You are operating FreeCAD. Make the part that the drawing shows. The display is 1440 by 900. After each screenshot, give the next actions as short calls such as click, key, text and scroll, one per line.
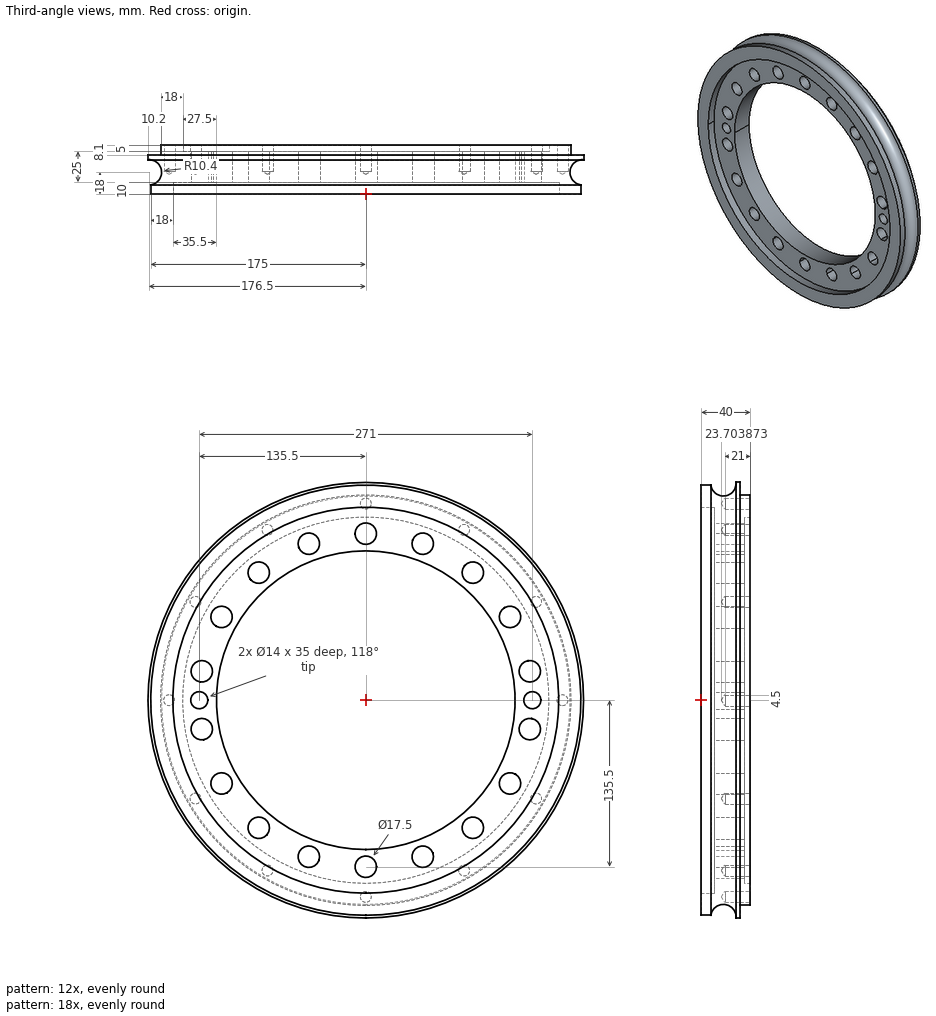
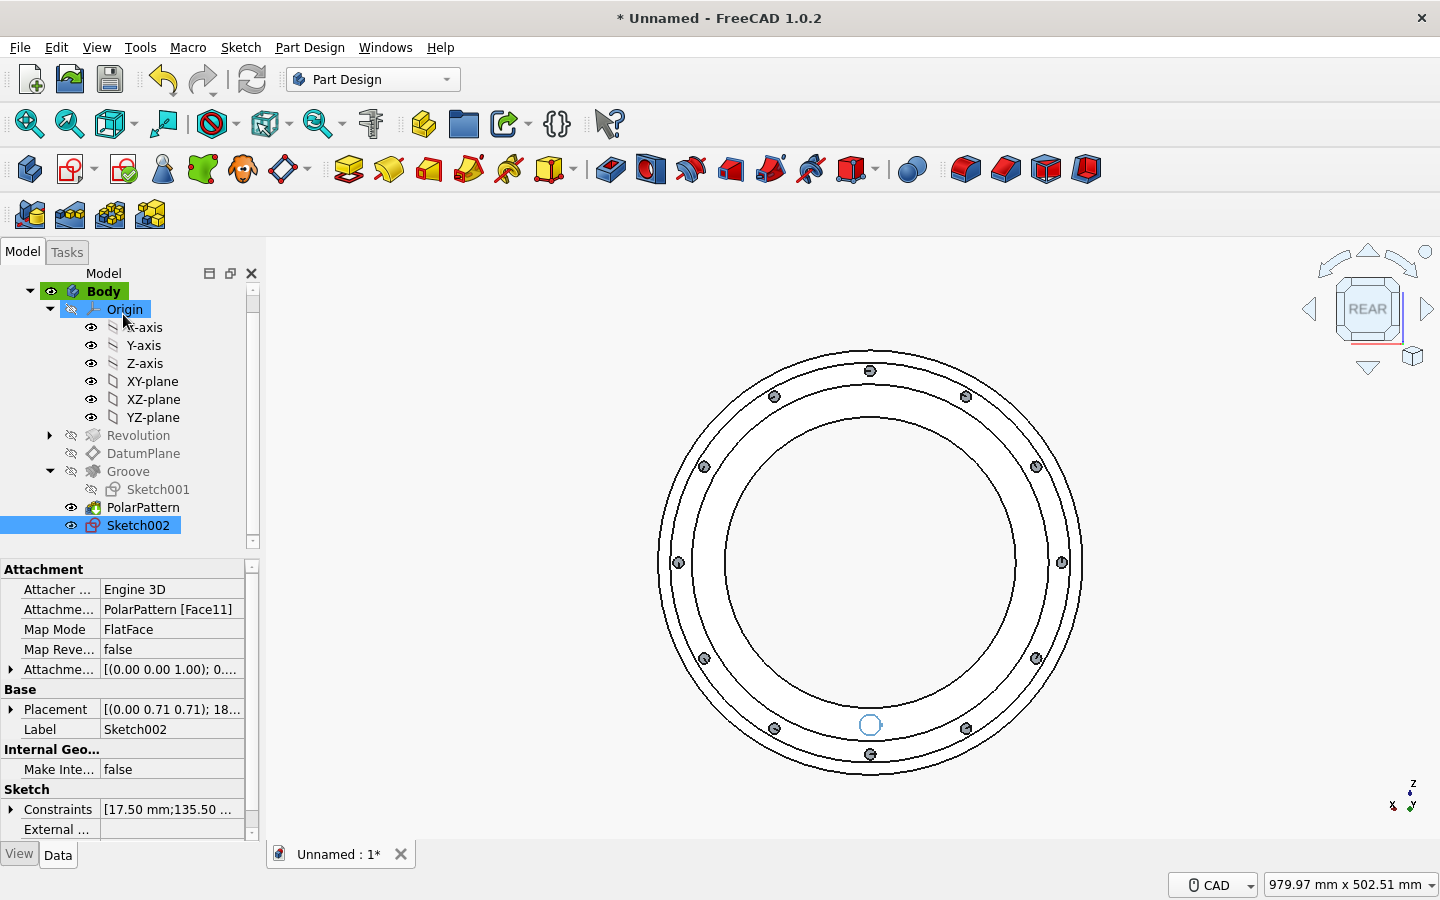
click(612, 170)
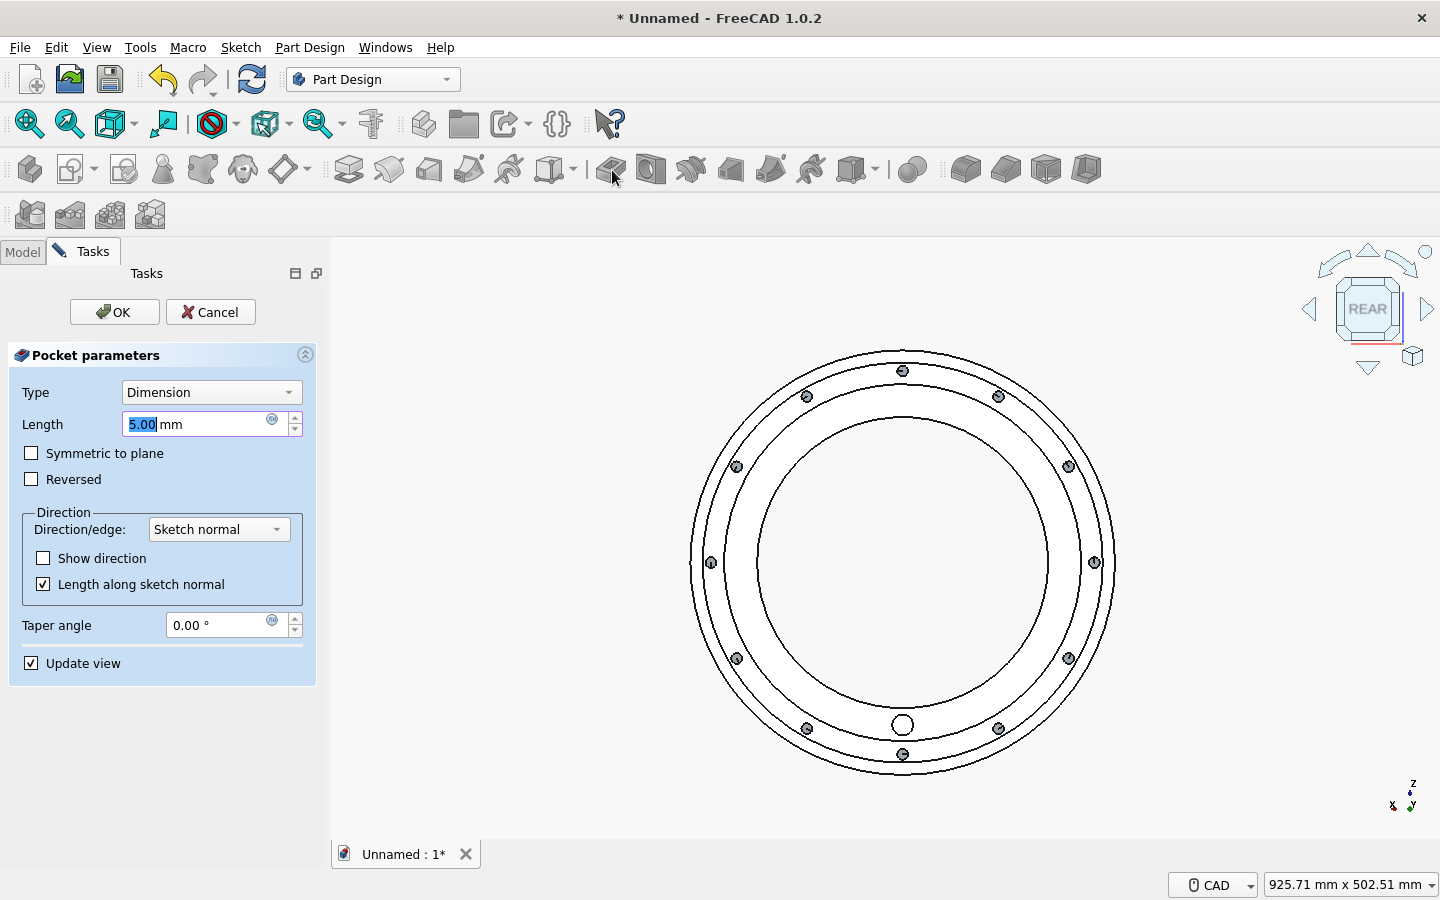
click(212, 392)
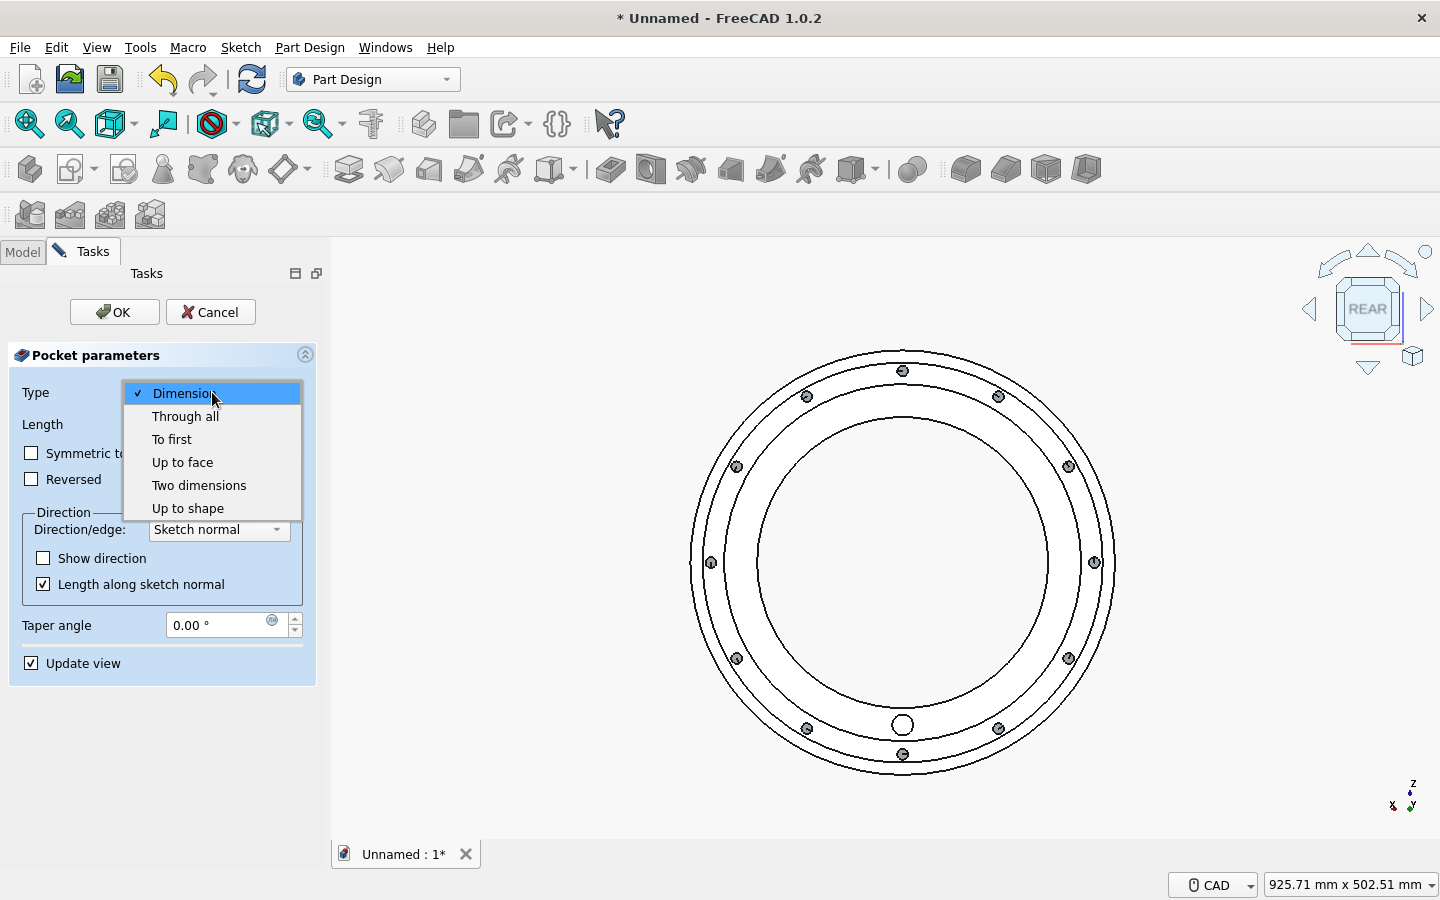
click(212, 416)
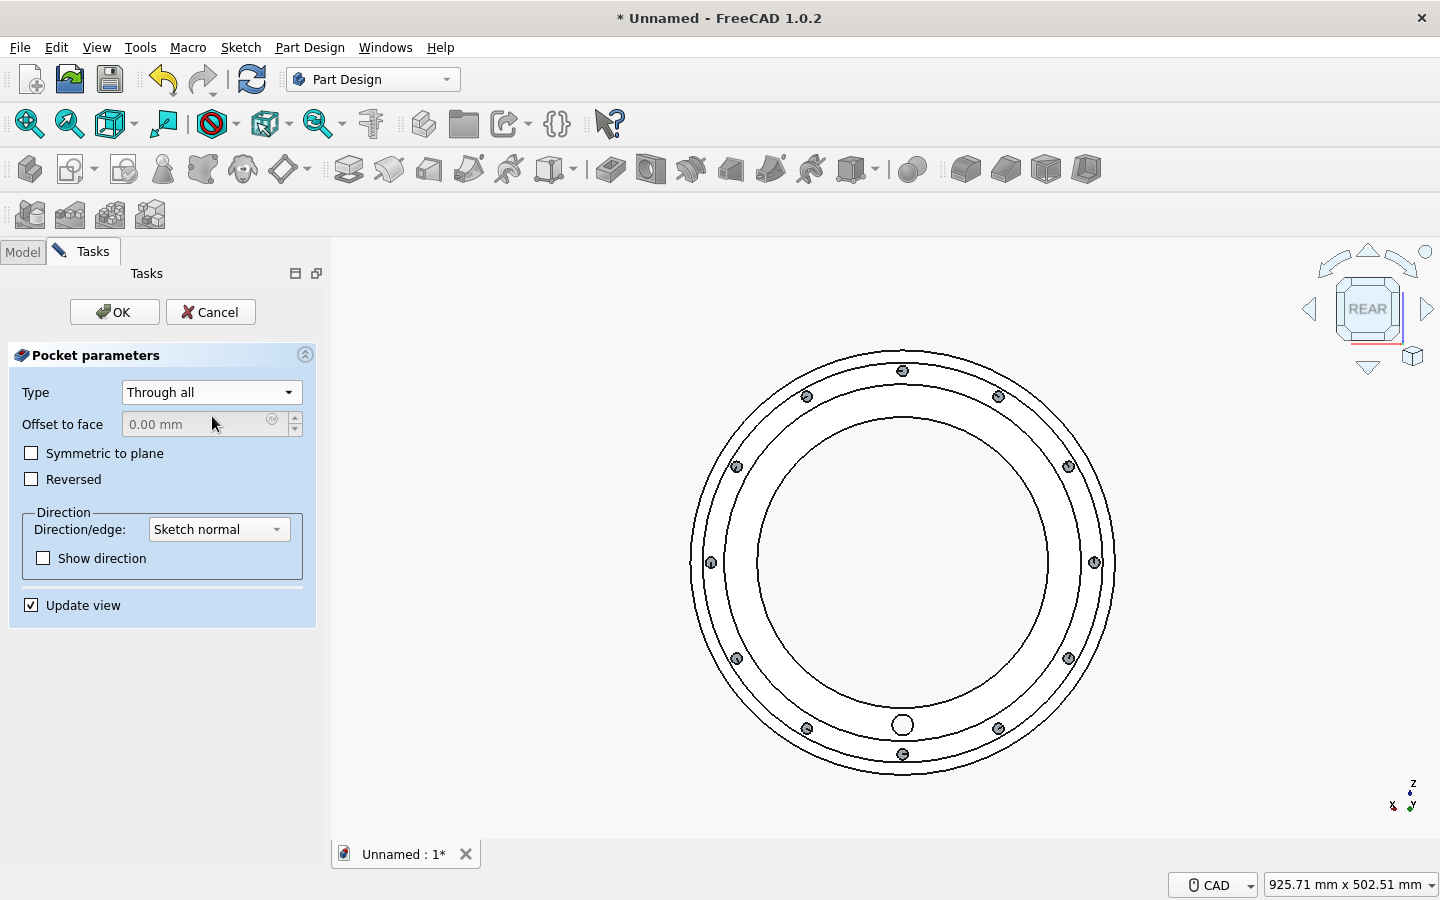
click(115, 312)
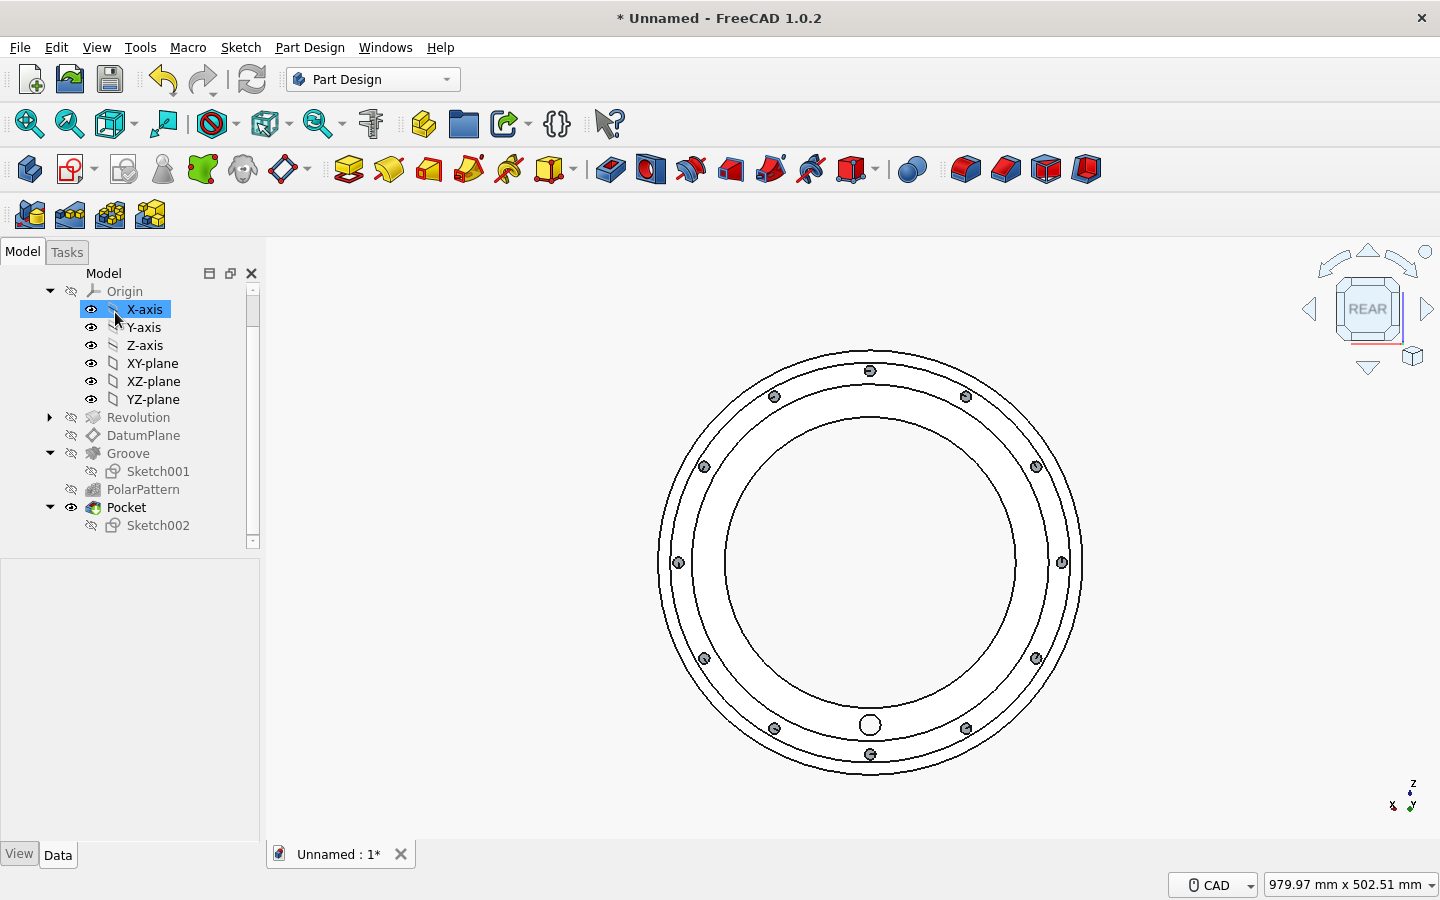
click(116, 507)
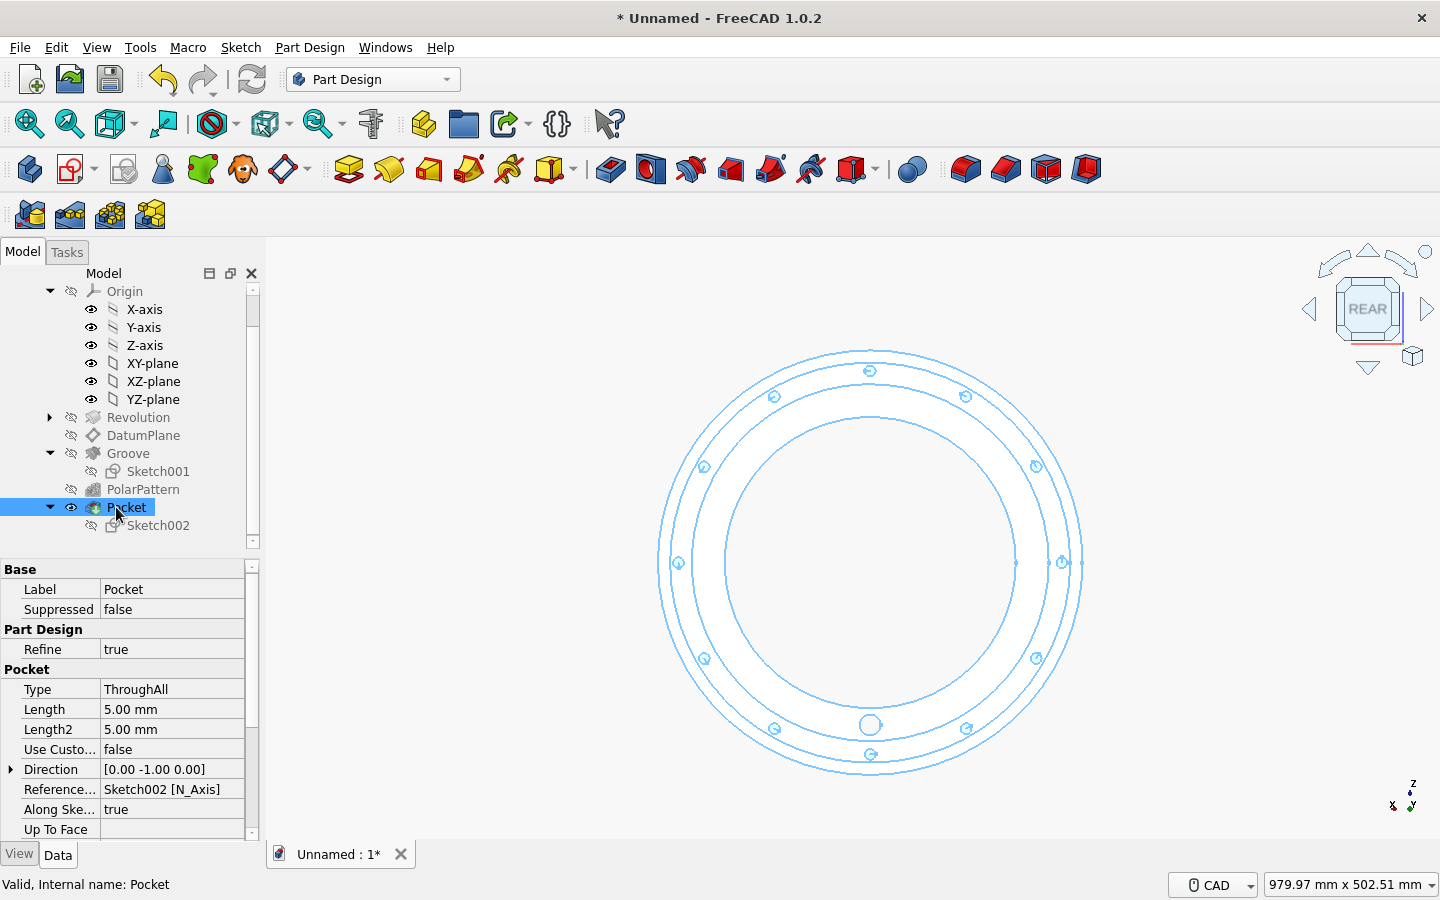
click(110, 214)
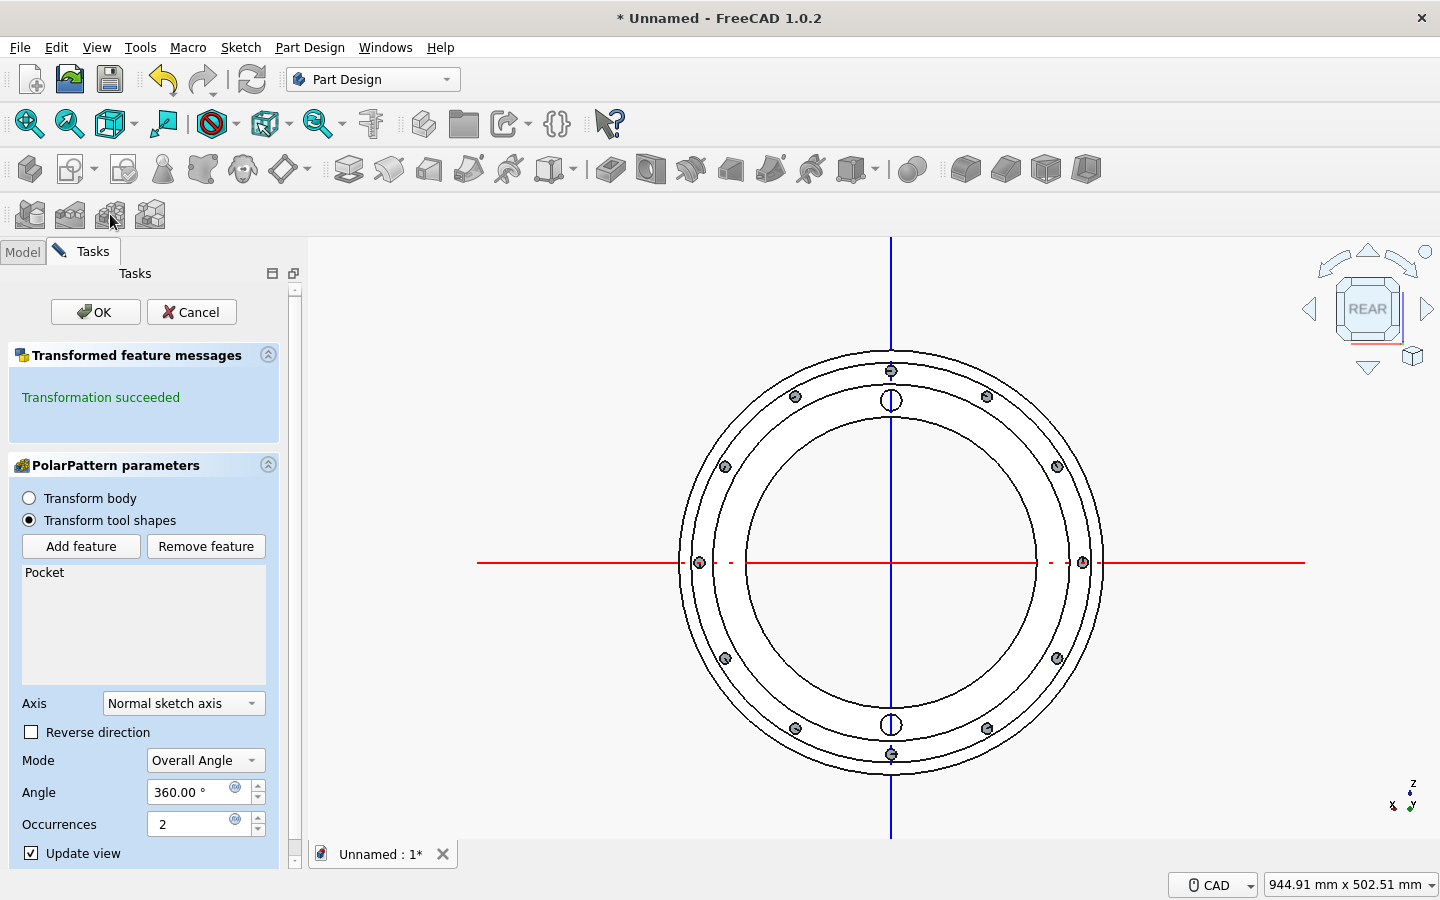
click(184, 704)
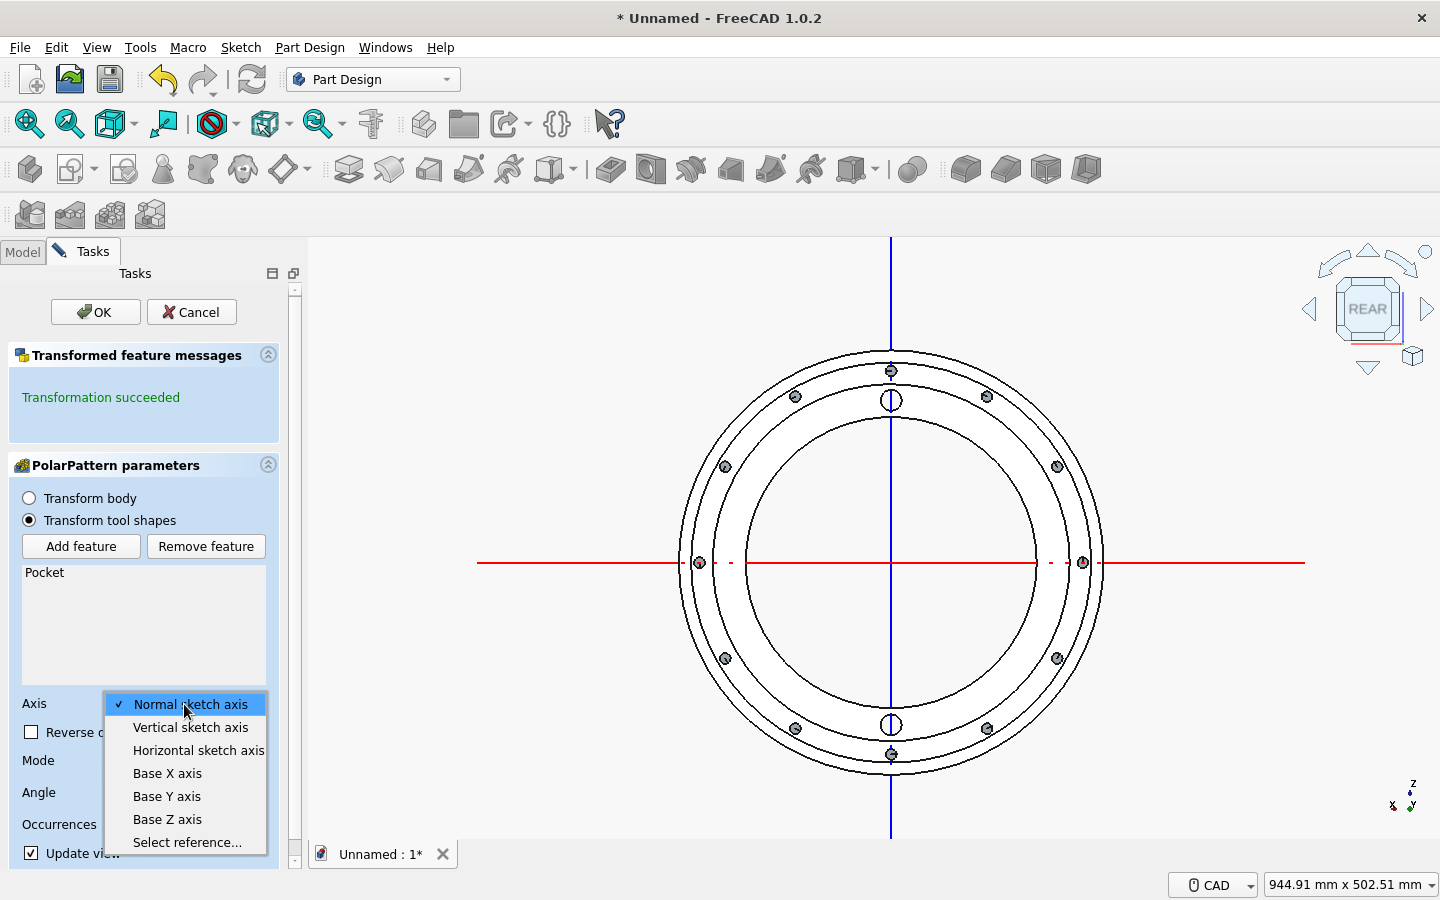
click(184, 796)